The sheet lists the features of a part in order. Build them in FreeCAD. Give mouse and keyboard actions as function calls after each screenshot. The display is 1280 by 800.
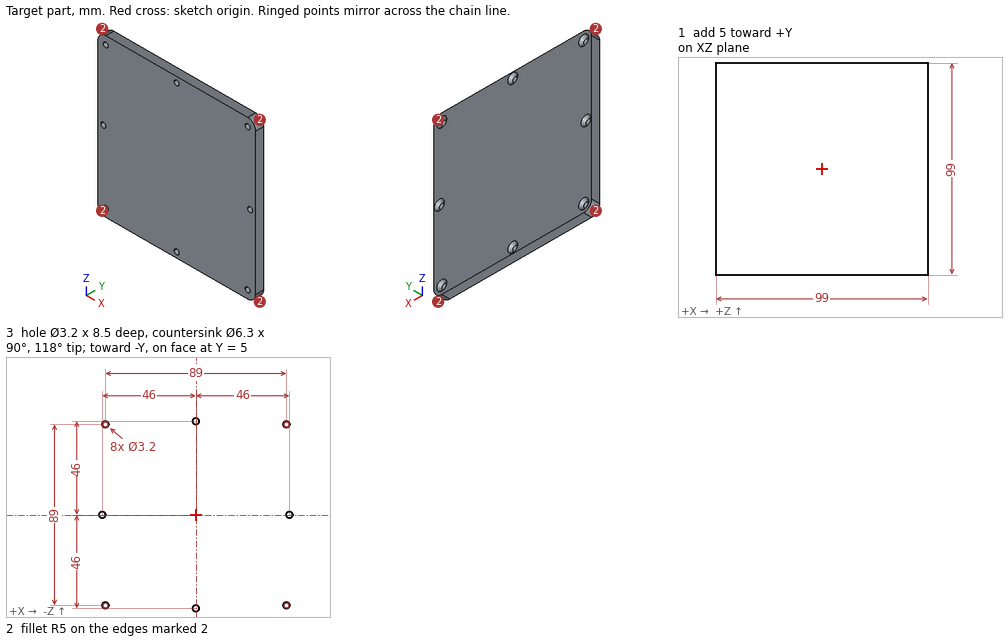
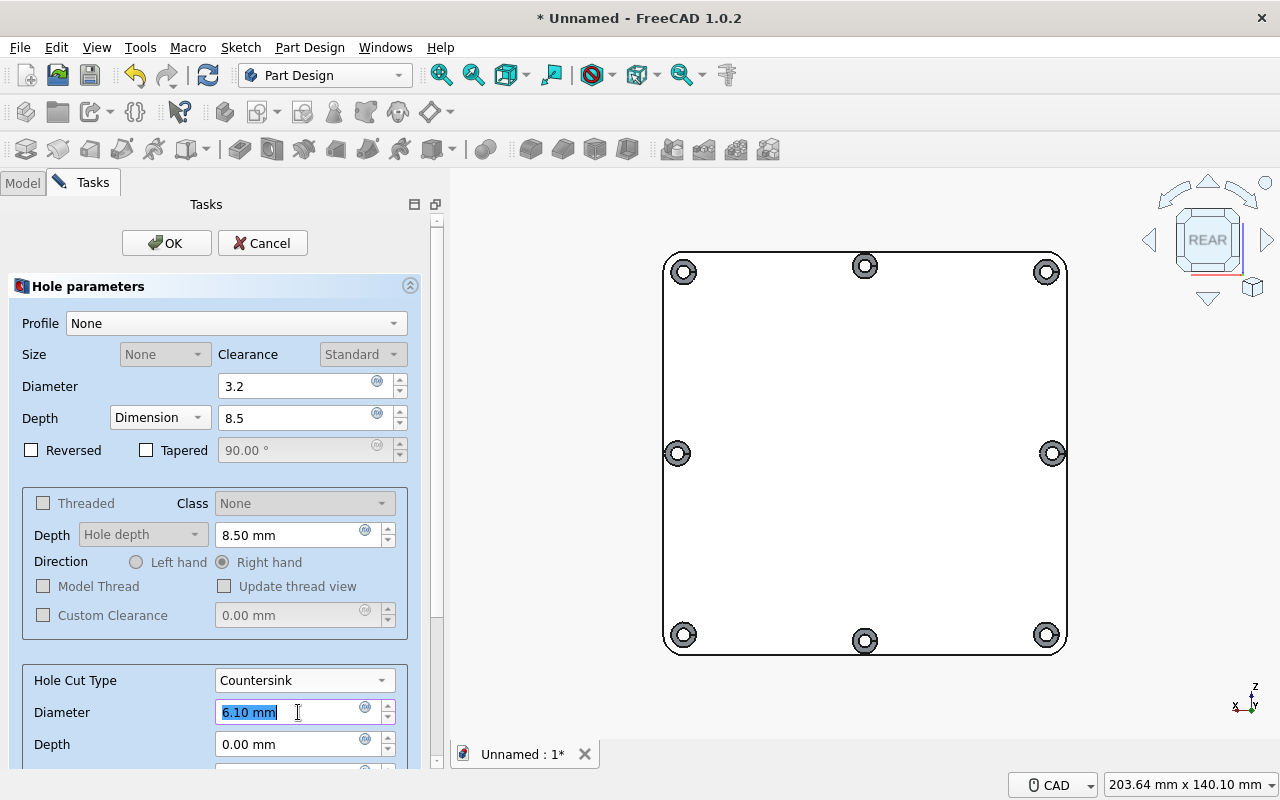
text(6.3)
key(Tab)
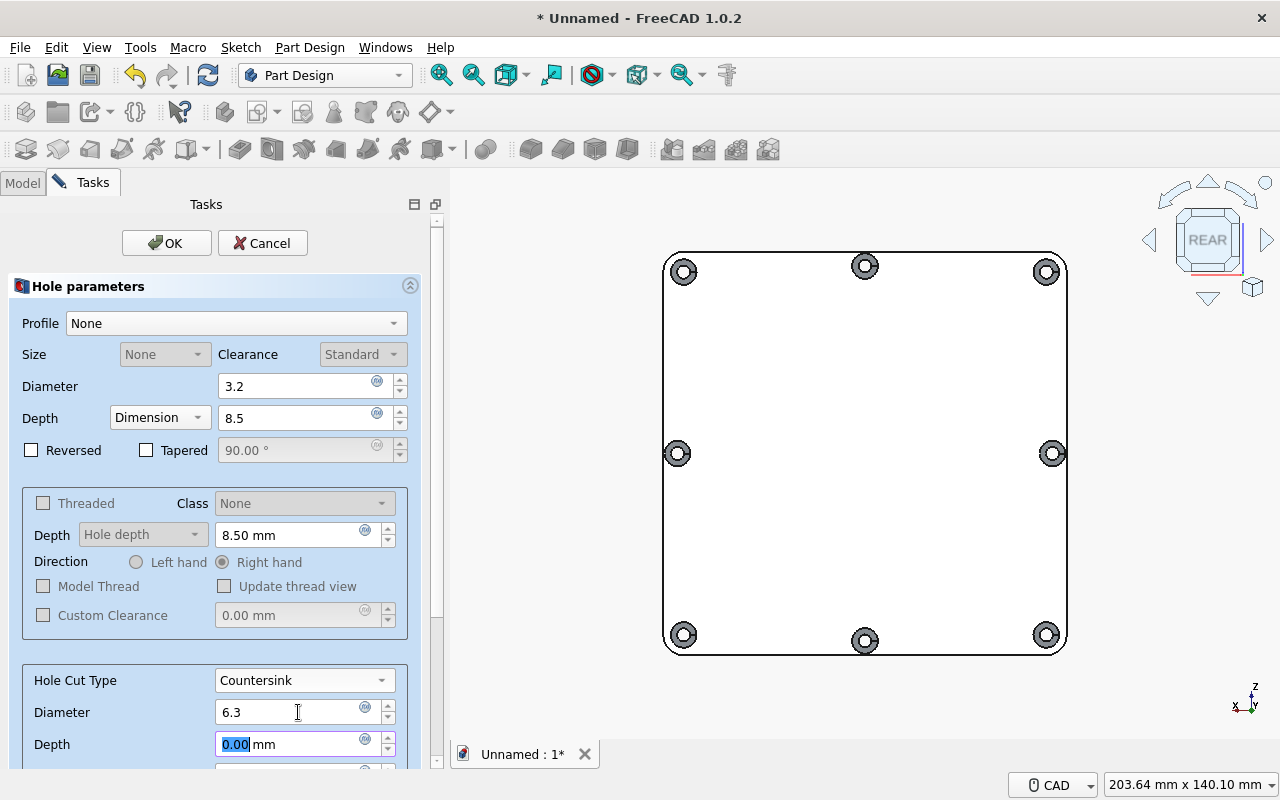
click(167, 243)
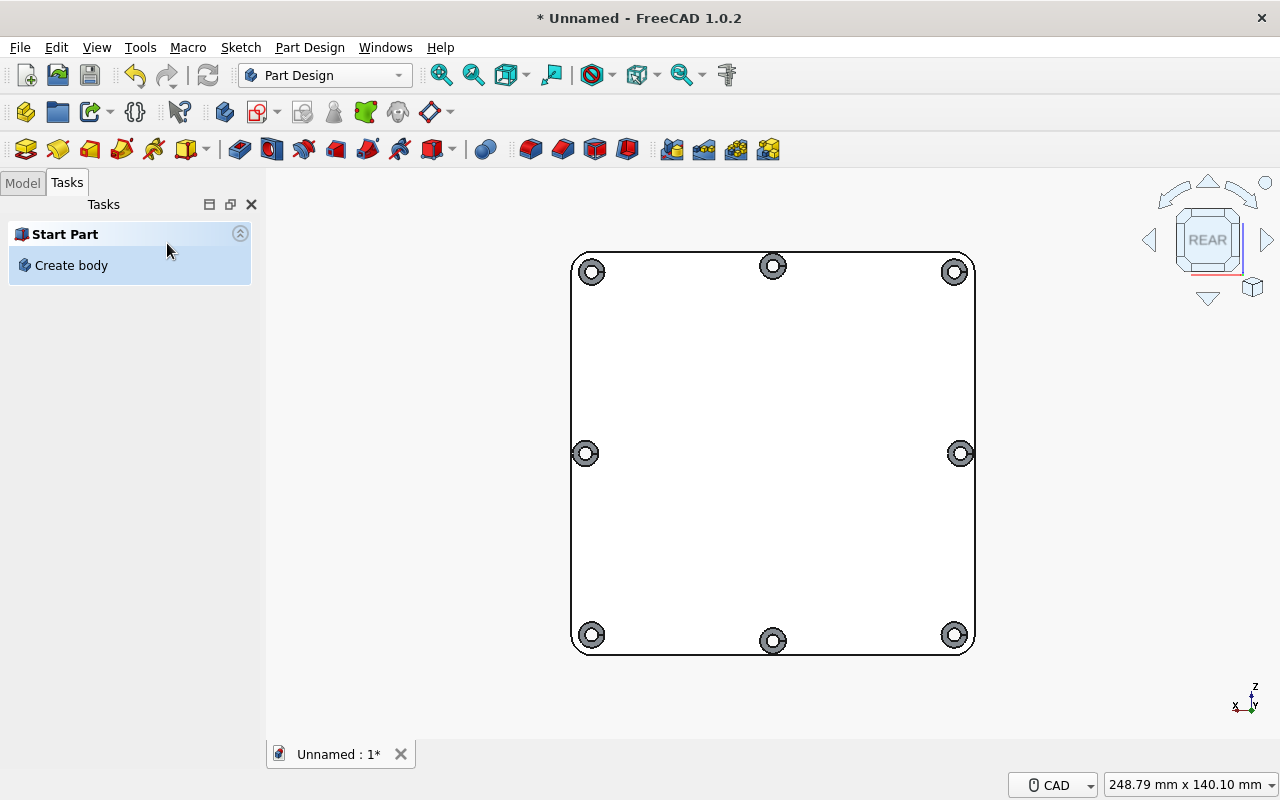
key(0)